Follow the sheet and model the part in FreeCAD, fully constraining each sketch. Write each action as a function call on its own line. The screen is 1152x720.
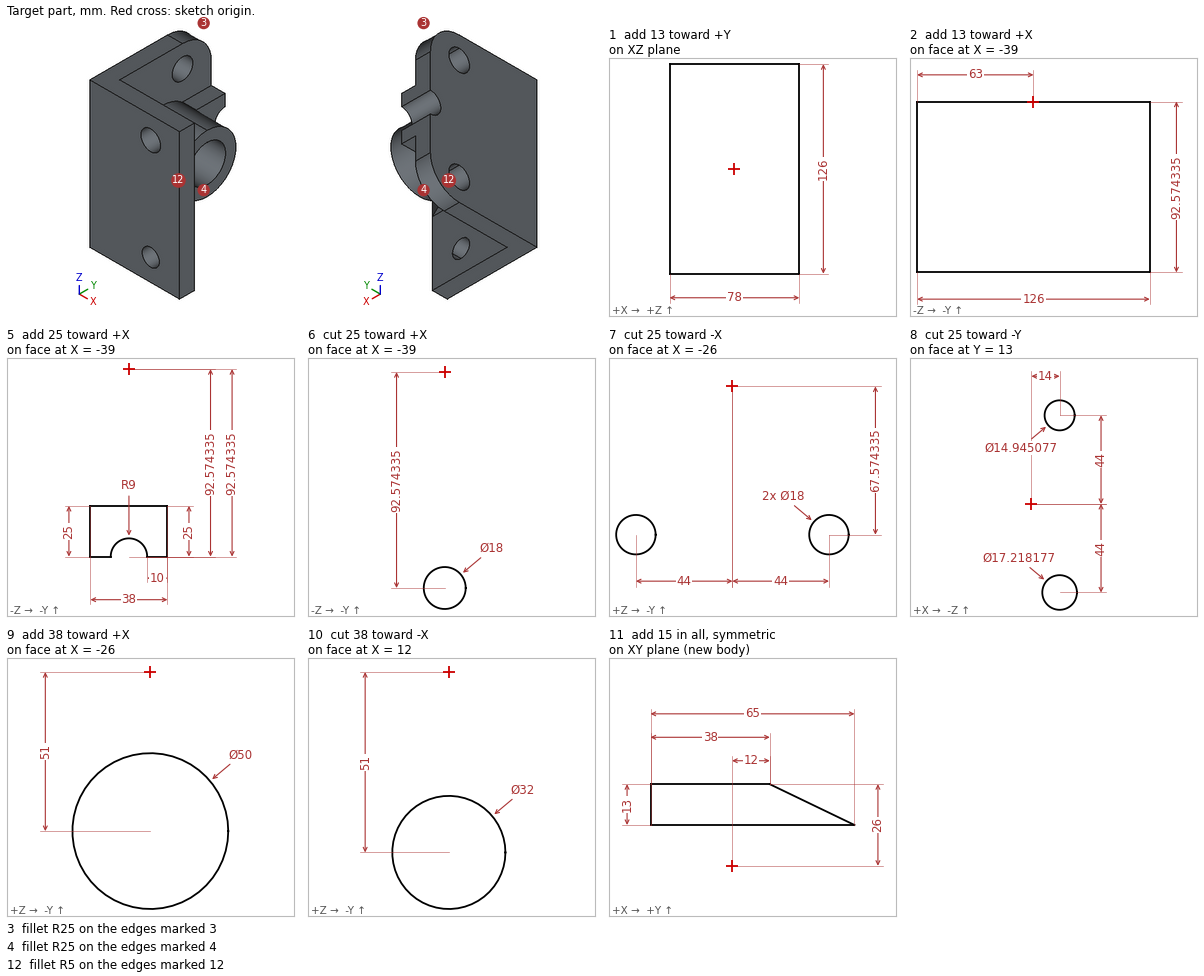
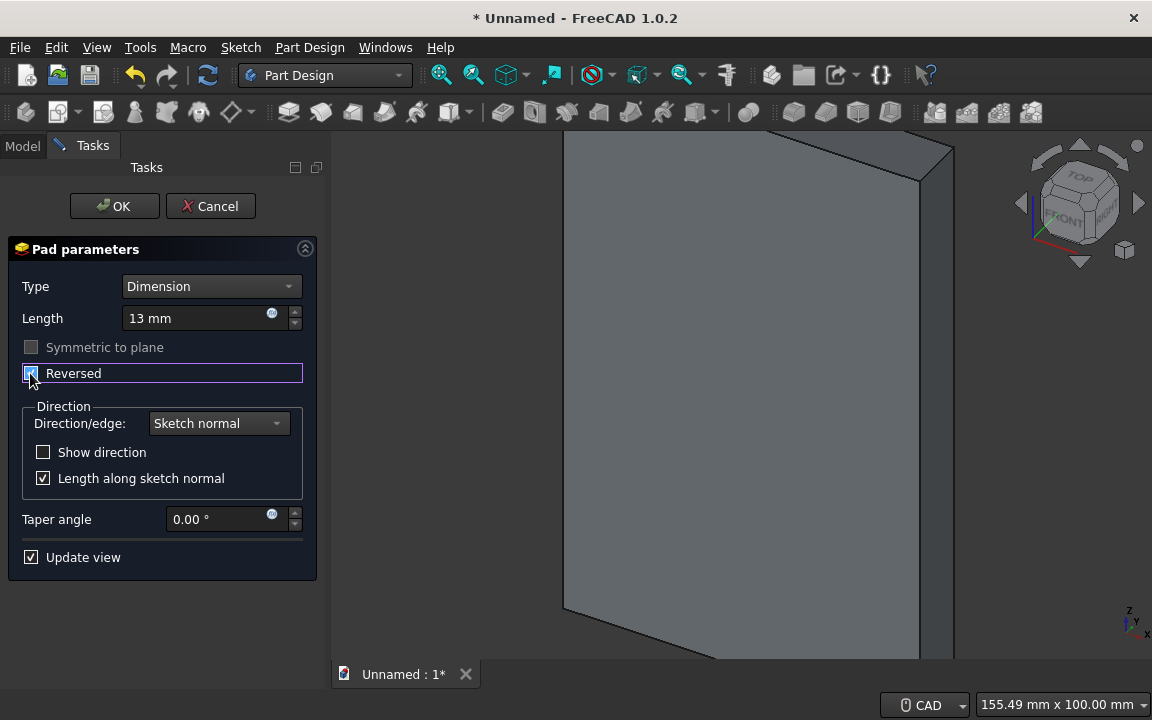
click(115, 206)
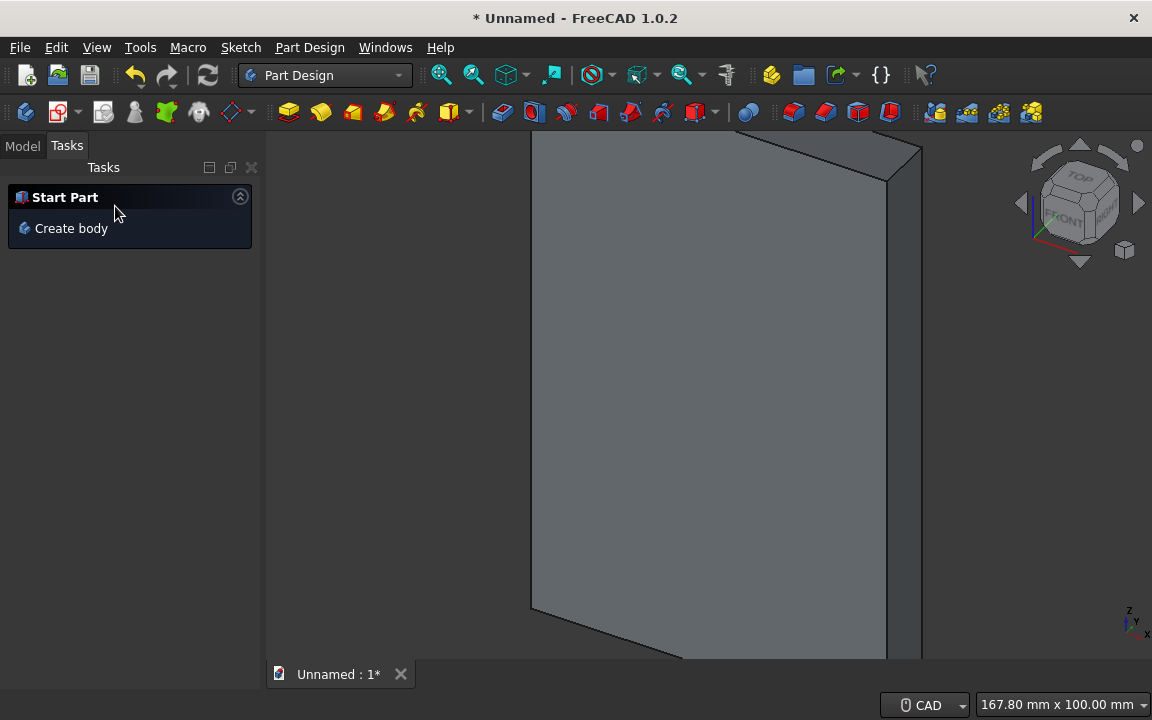
key(v)
key(f)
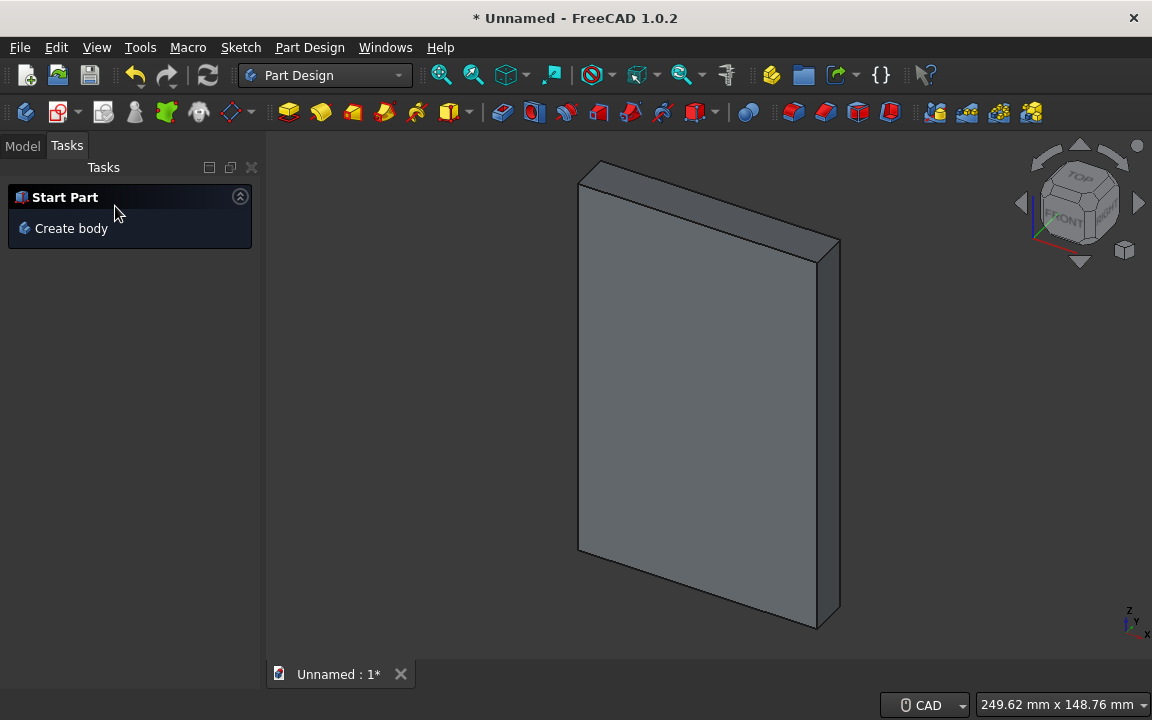
key(6)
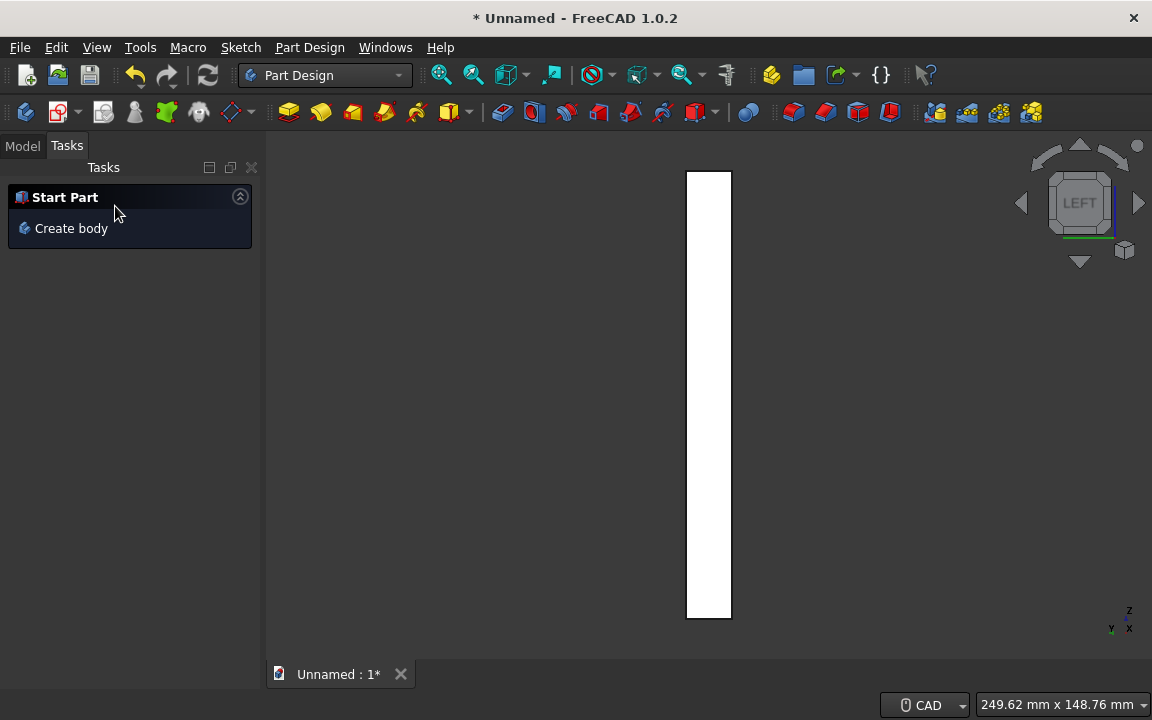
click(709, 266)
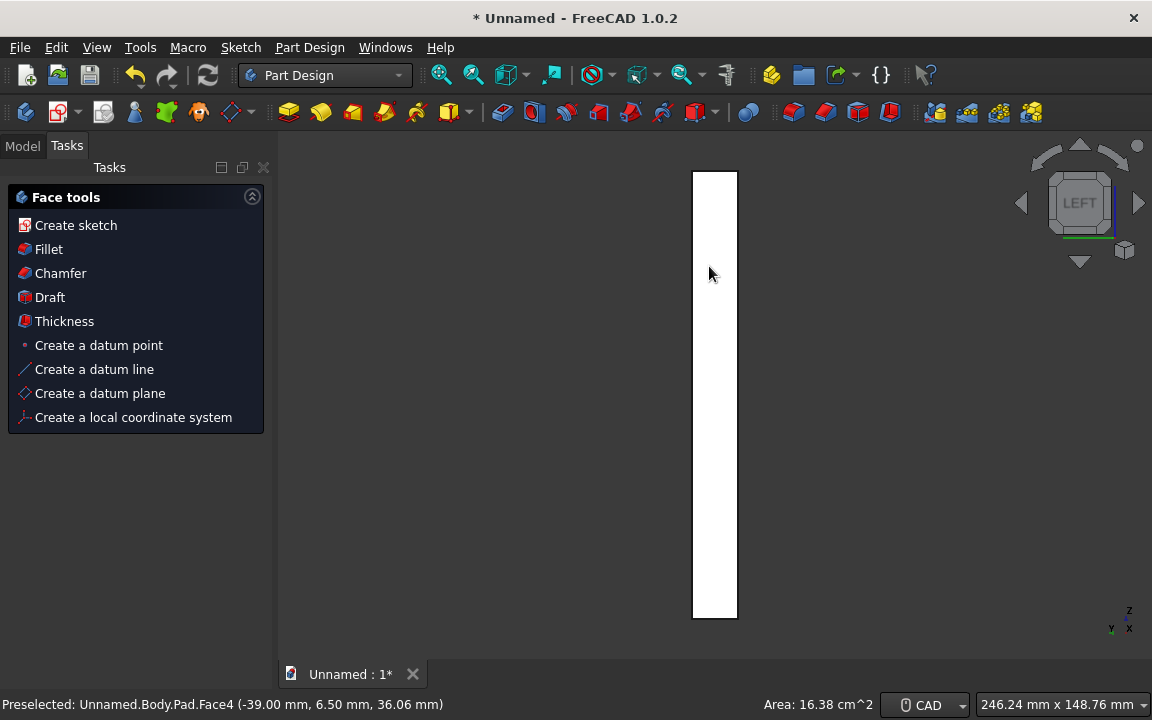
click(58, 112)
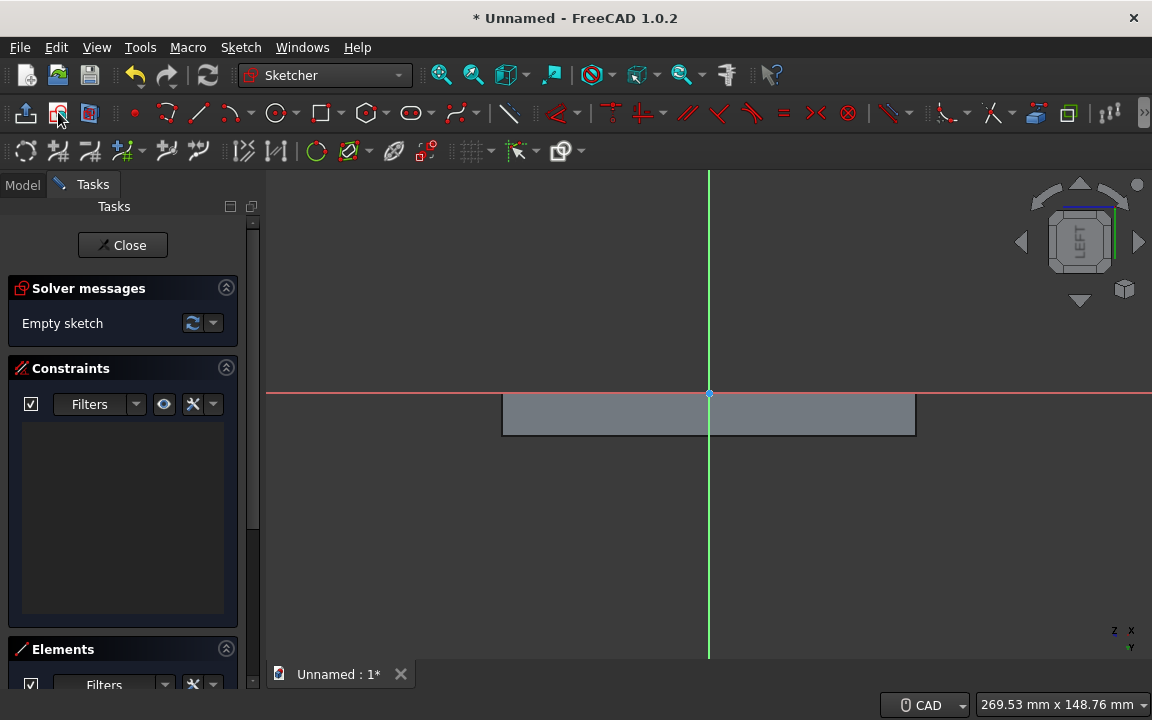
scroll(501, 198, down, 2)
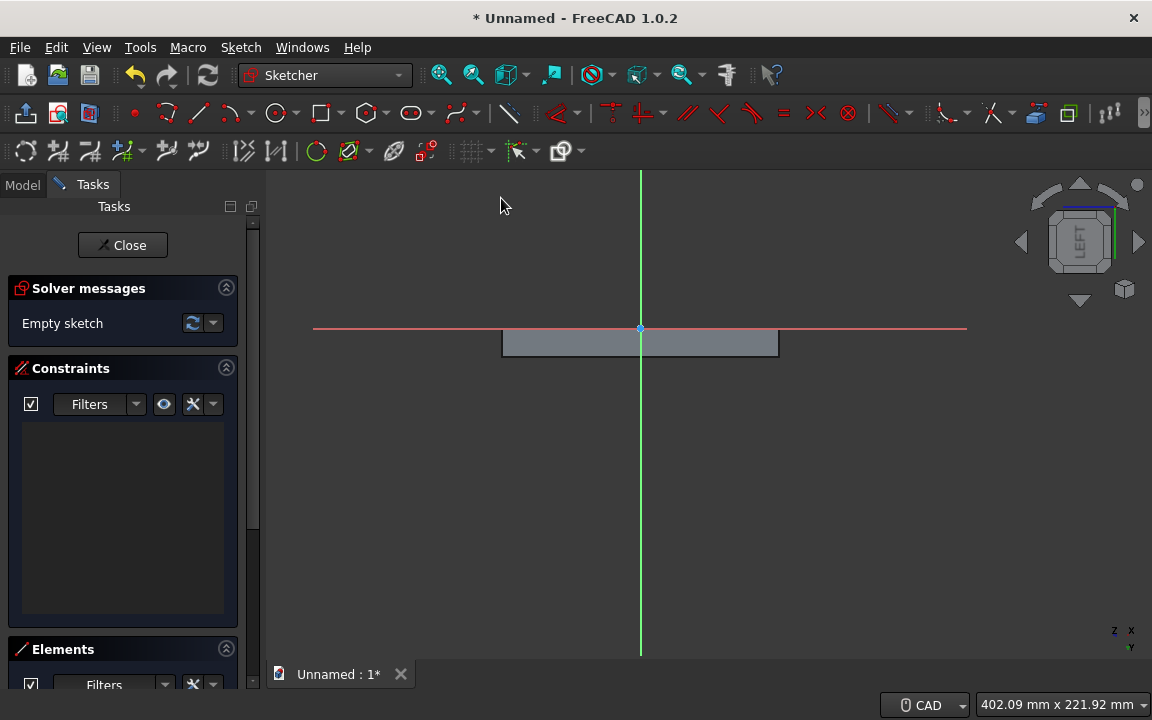
scroll(641, 464, up, 2)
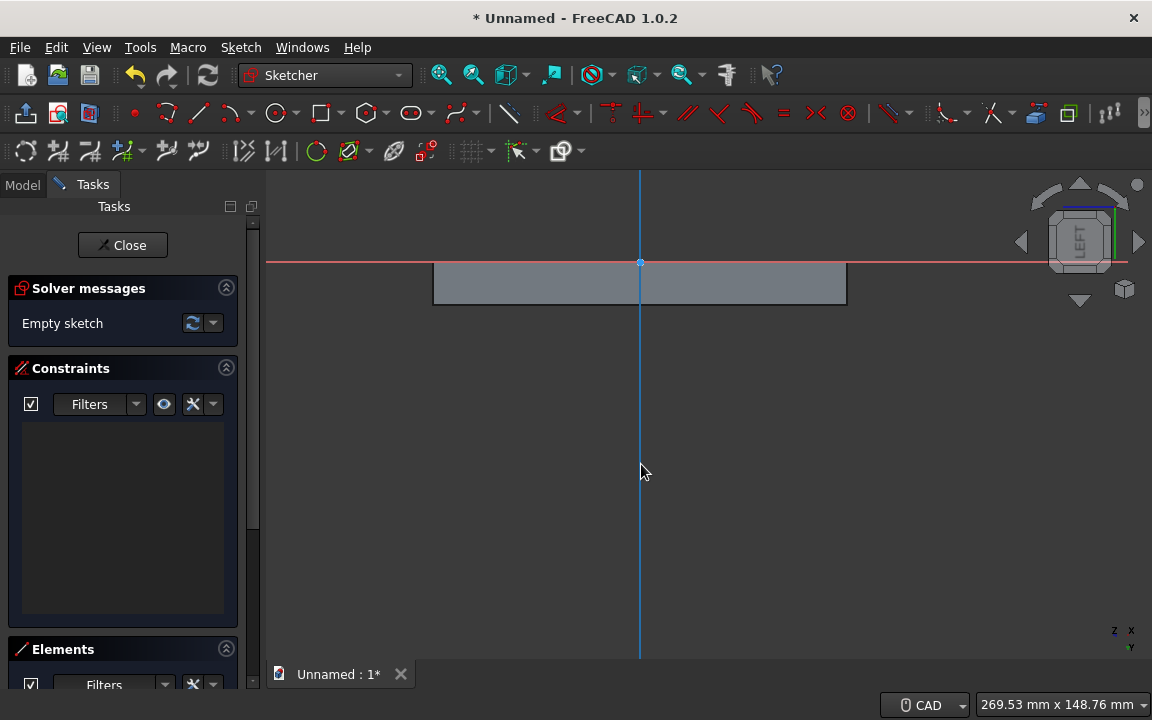
key(g)
key(r)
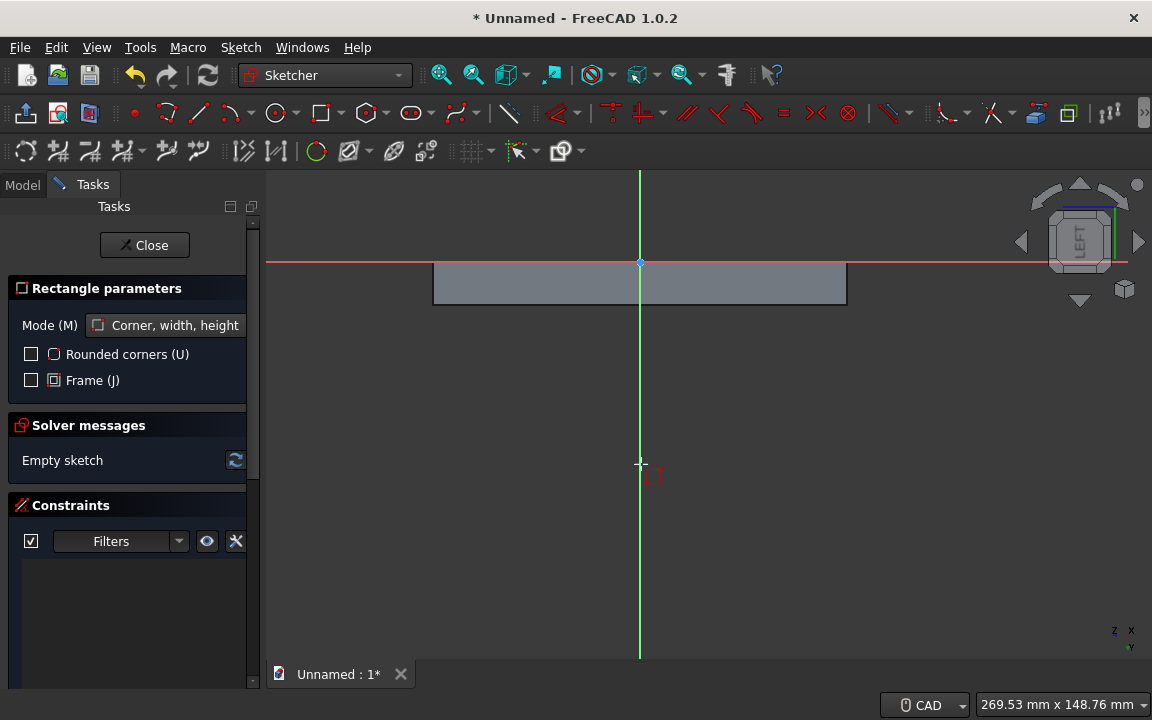
click(433, 262)
move(847, 566)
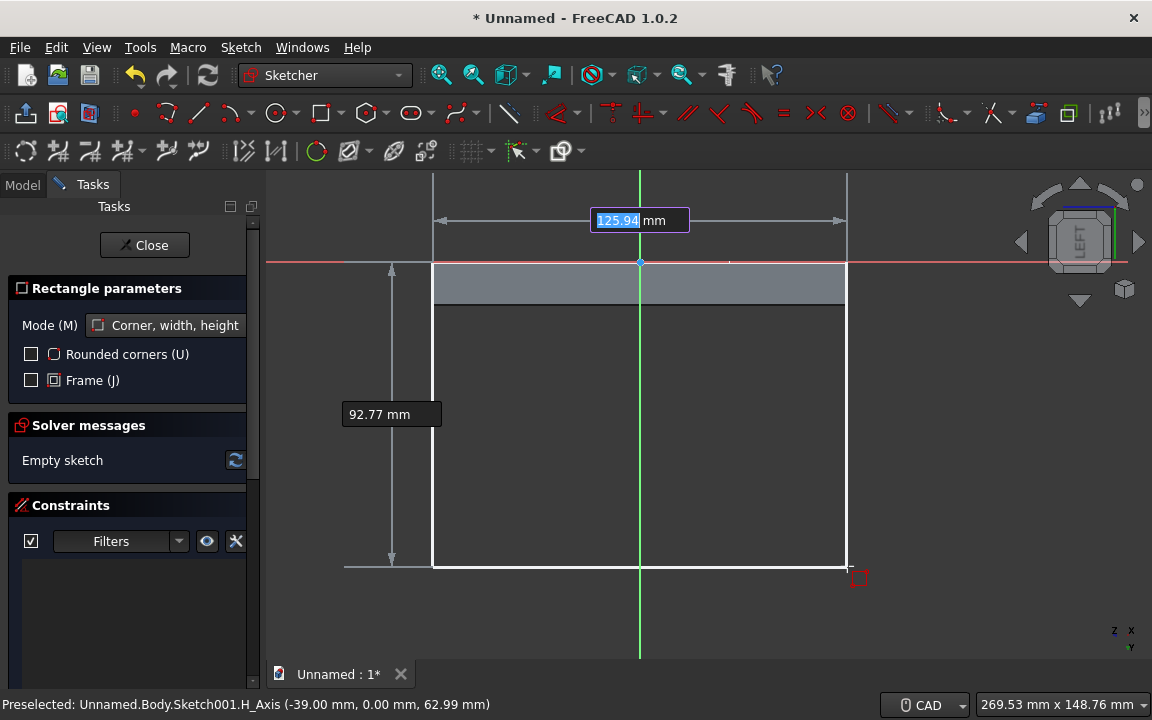
text(126)
key(Tab)
text(92.574335)
key(Return)
key(Escape)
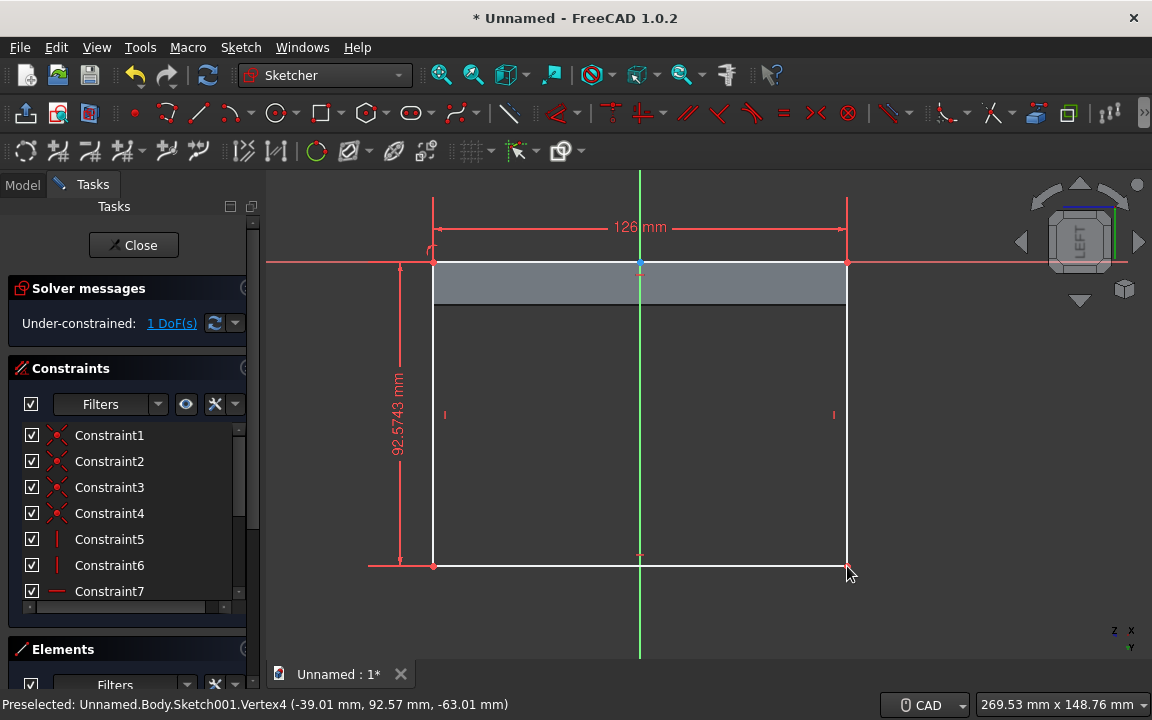
click(433, 262)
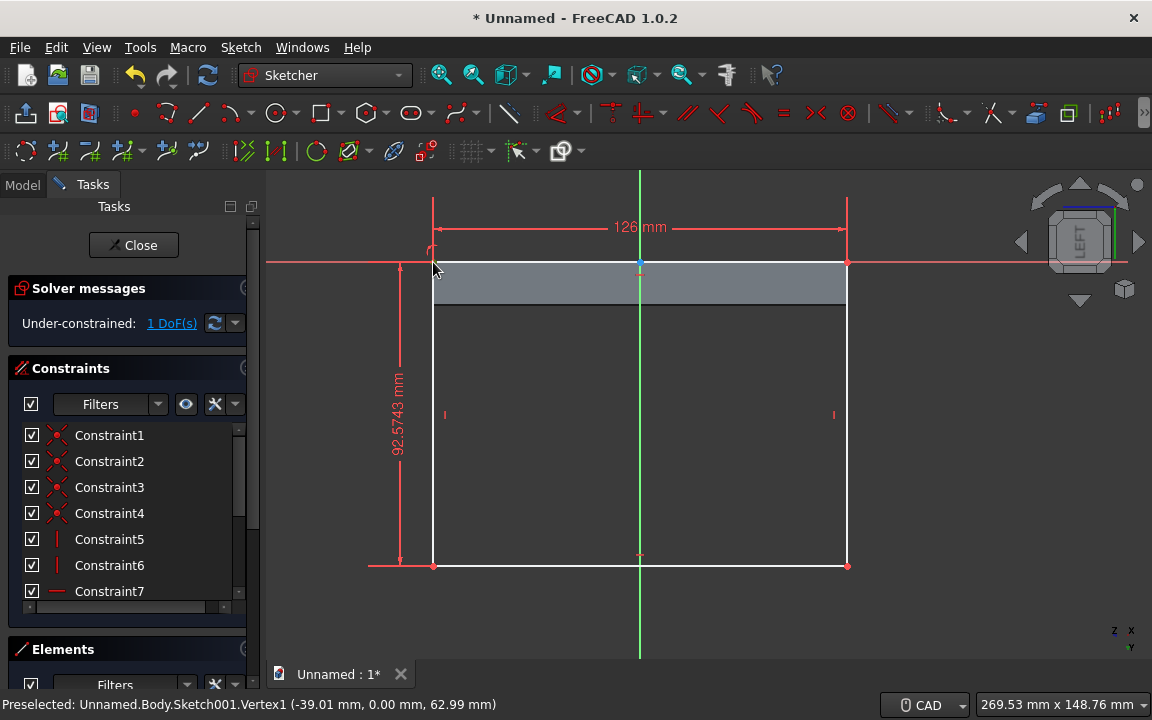
key(l)